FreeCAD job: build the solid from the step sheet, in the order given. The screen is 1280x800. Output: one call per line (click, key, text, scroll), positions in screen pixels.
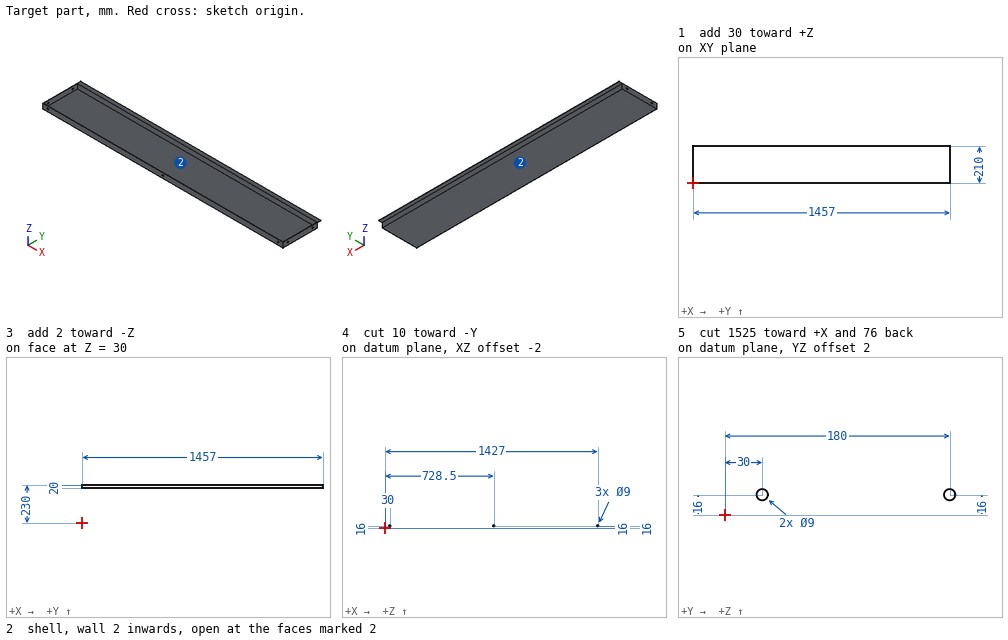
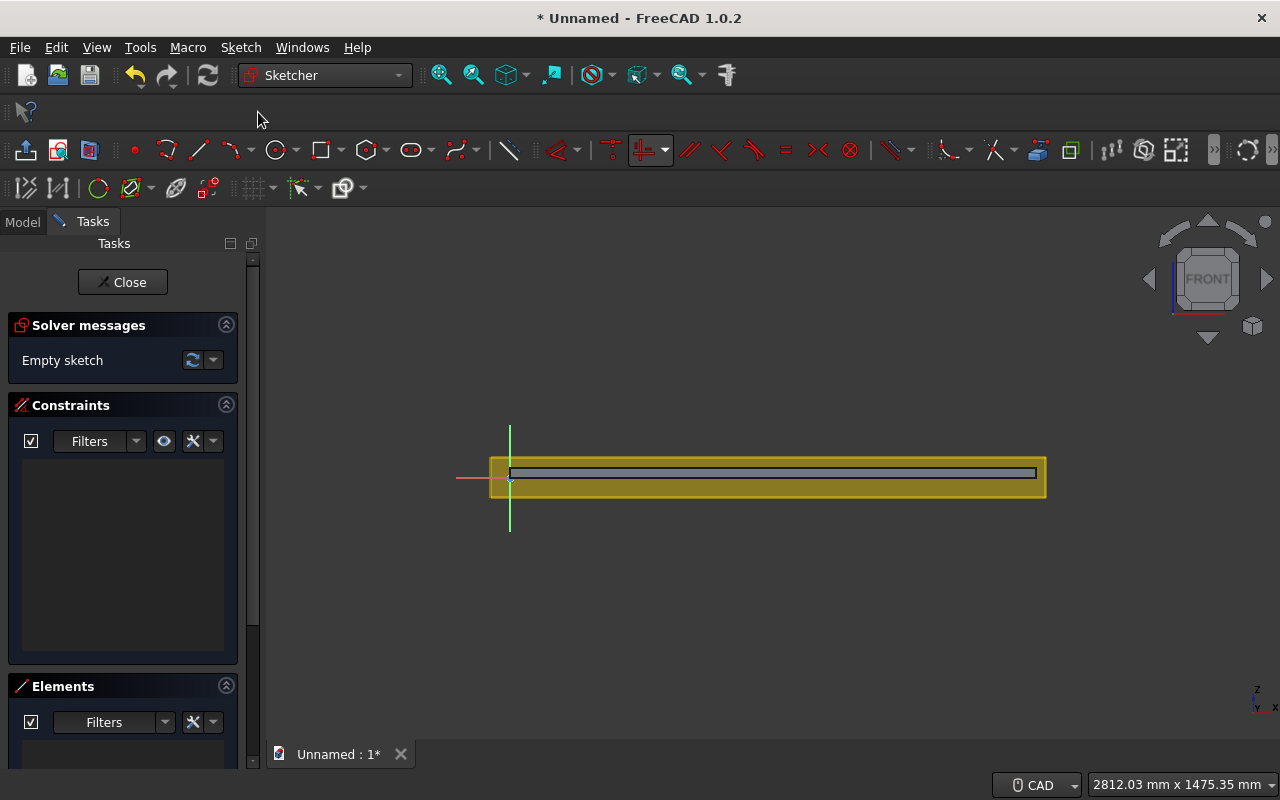
click(90, 150)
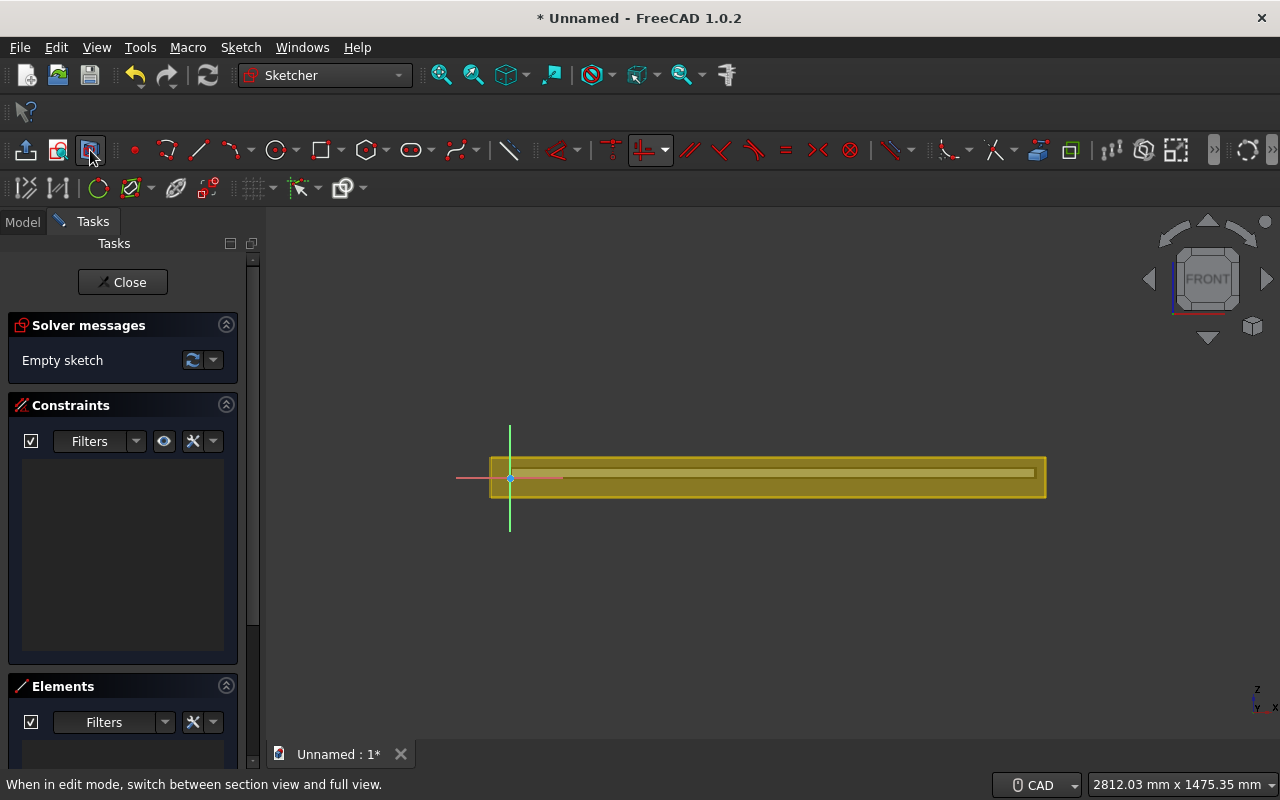
click(276, 150)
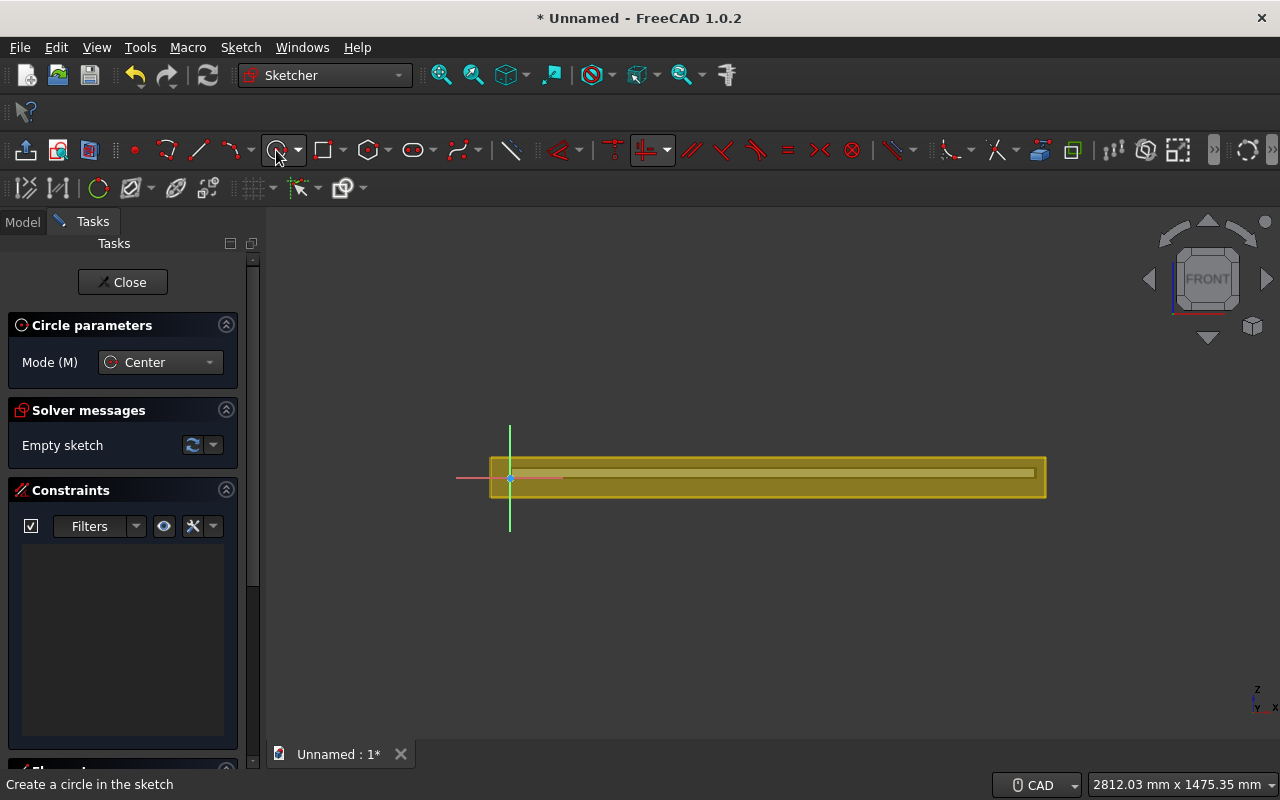
scroll(1025, 473, up, 14)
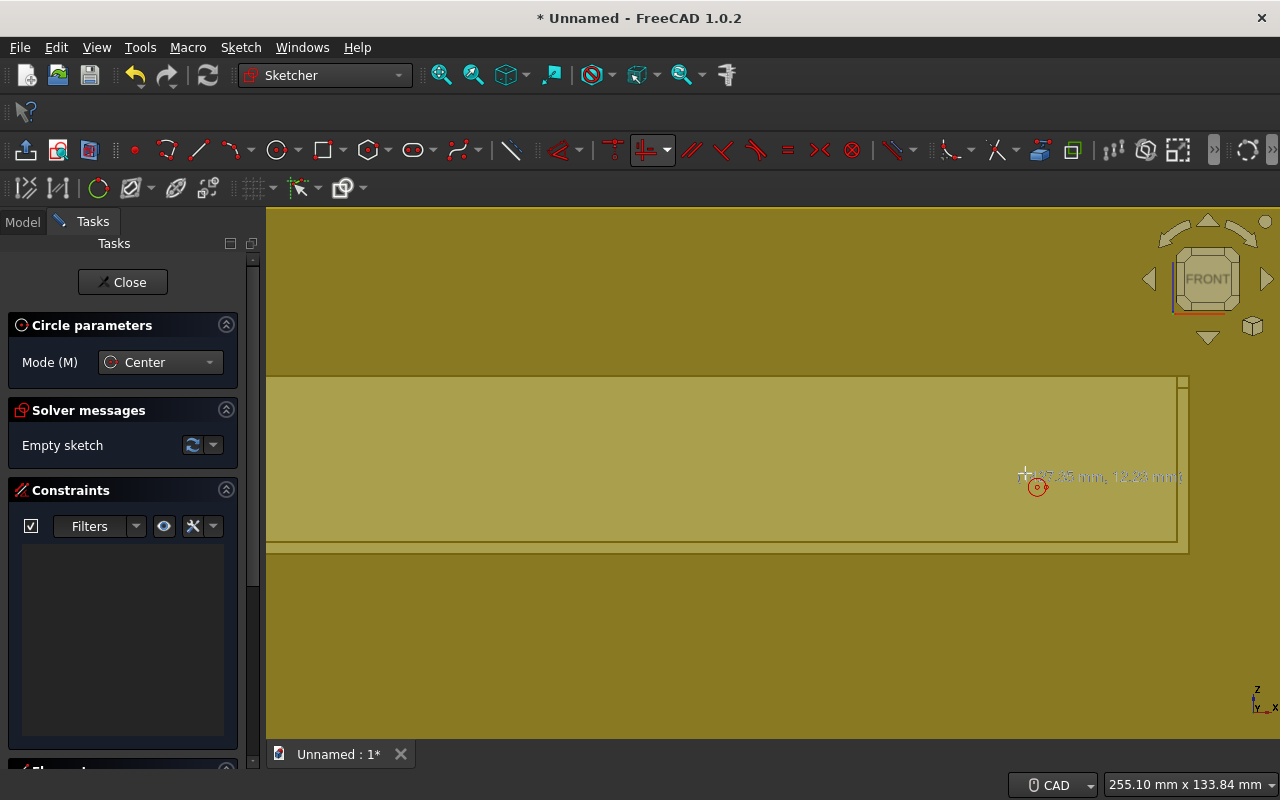
scroll(1018, 471, down, 13)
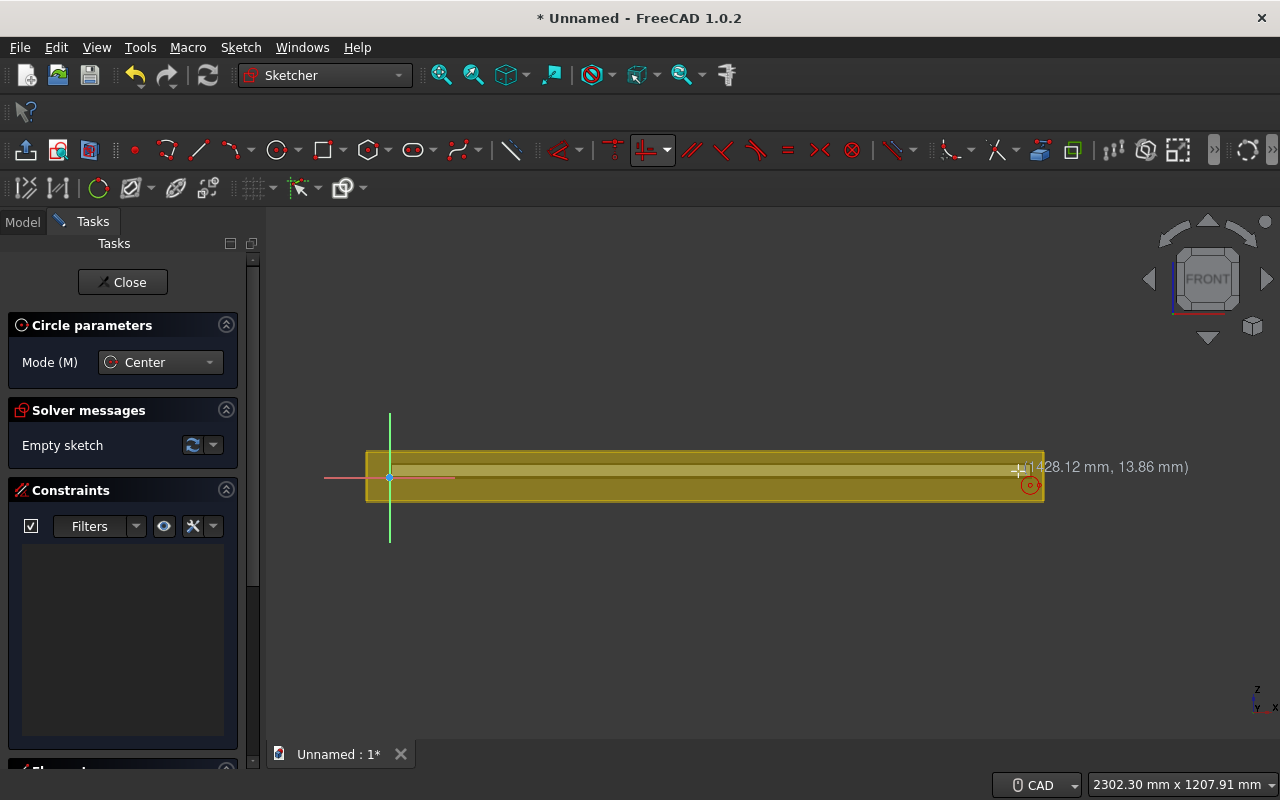
scroll(1018, 471, up, 5)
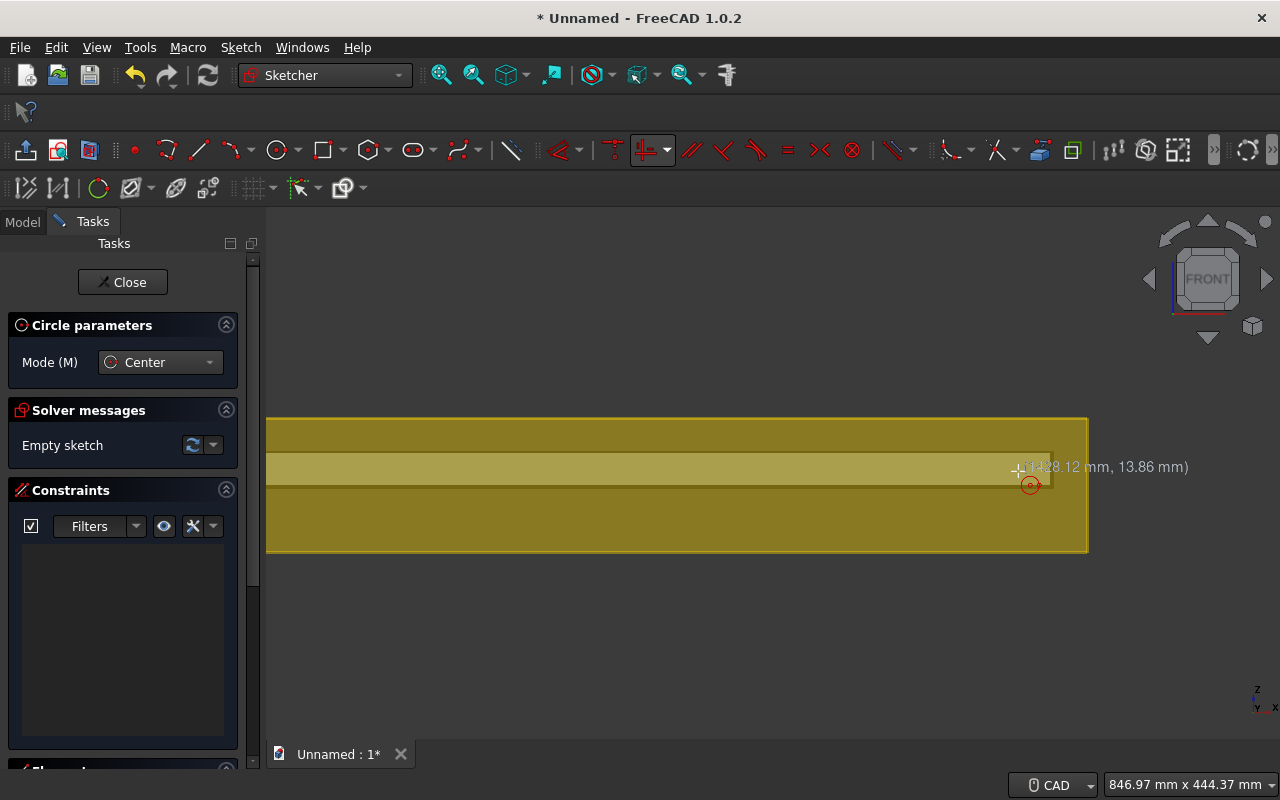
click(1017, 469)
move(1021, 465)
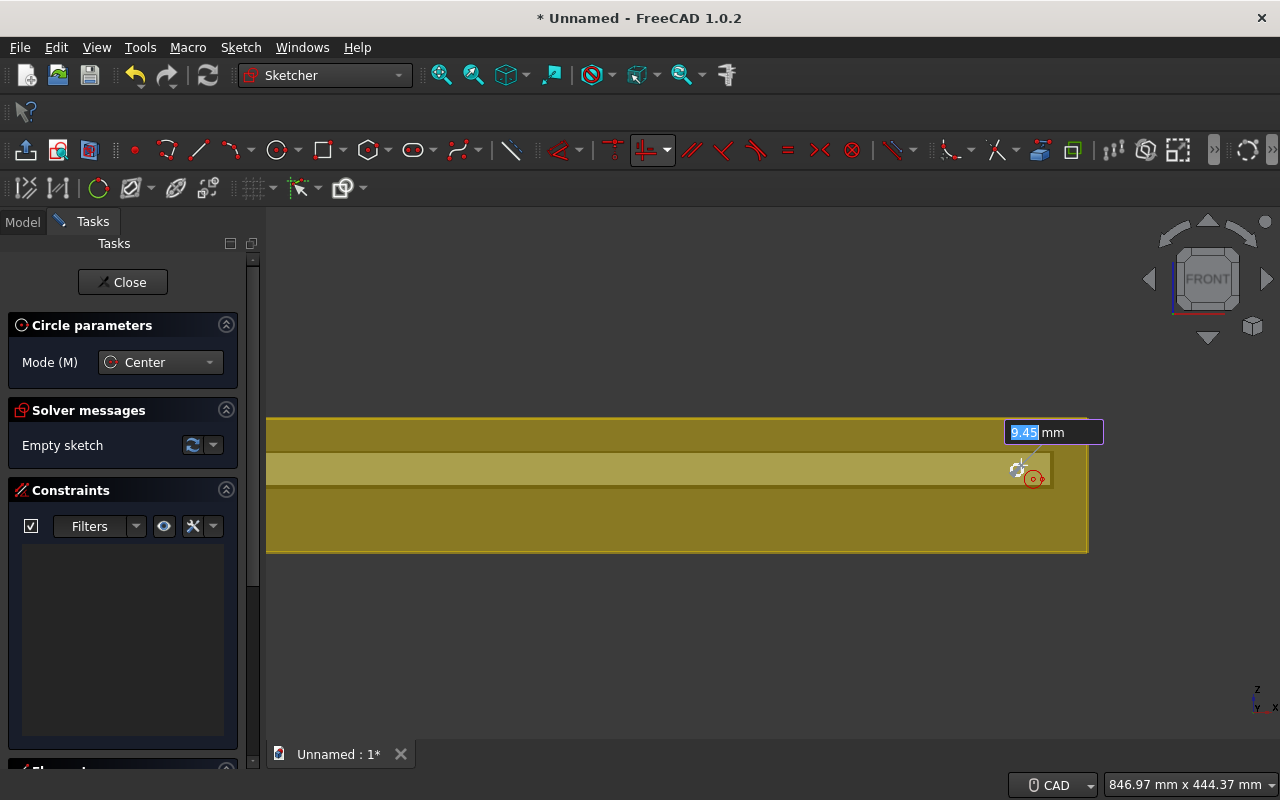
text(9)
key(Return)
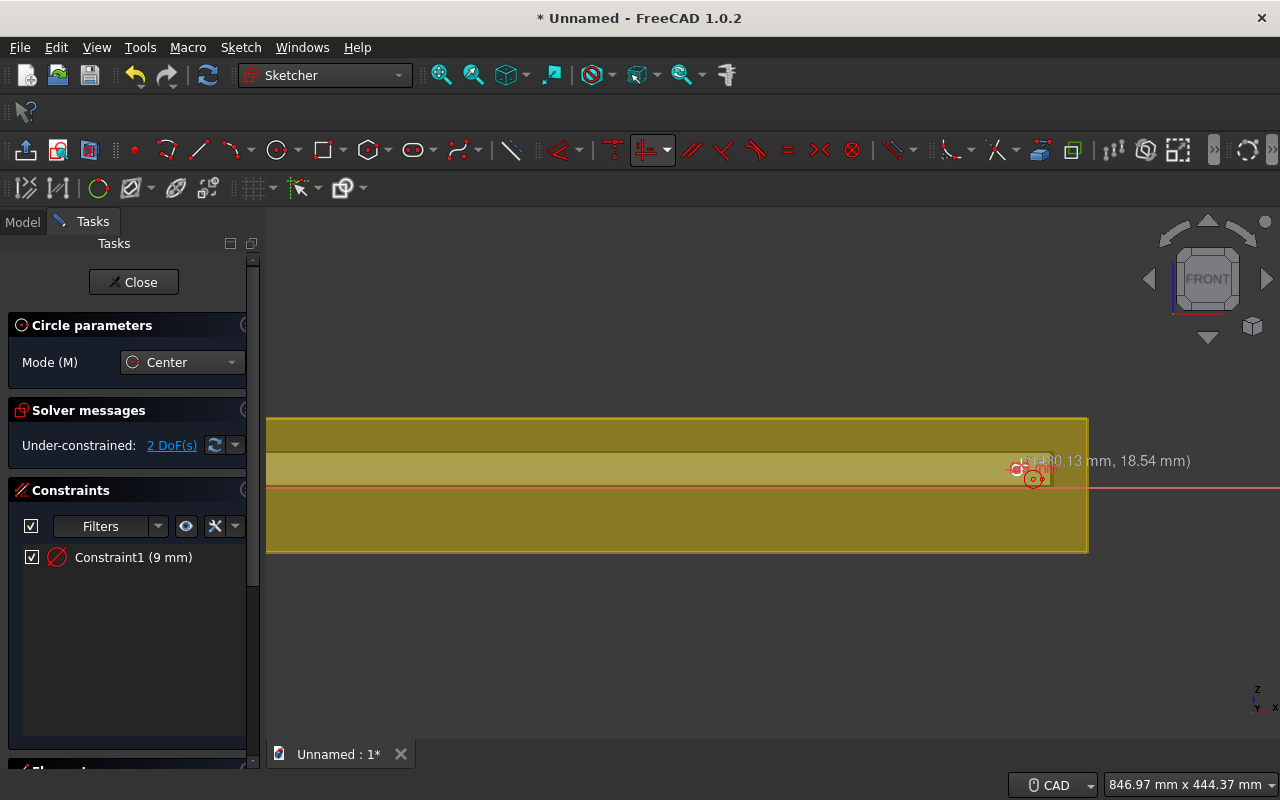
scroll(1018, 471, down, 5)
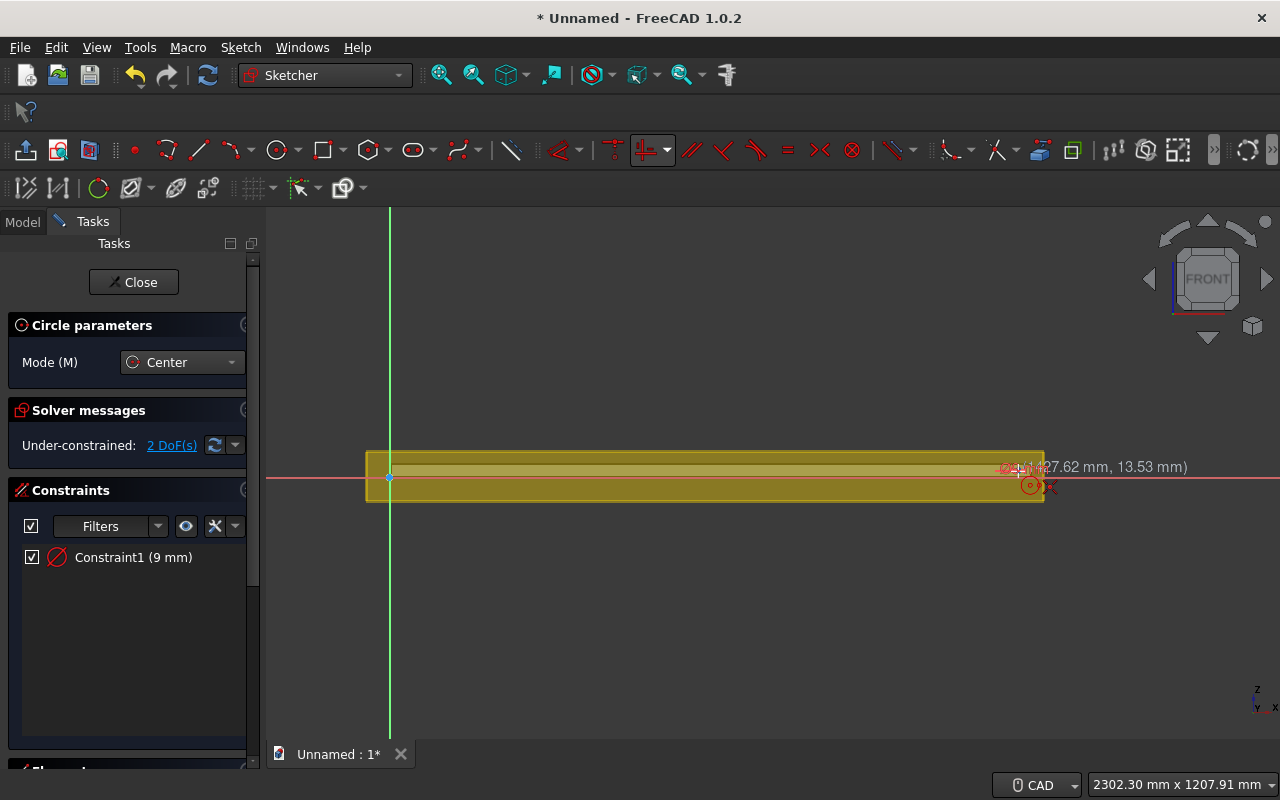
scroll(711, 471, up, 13)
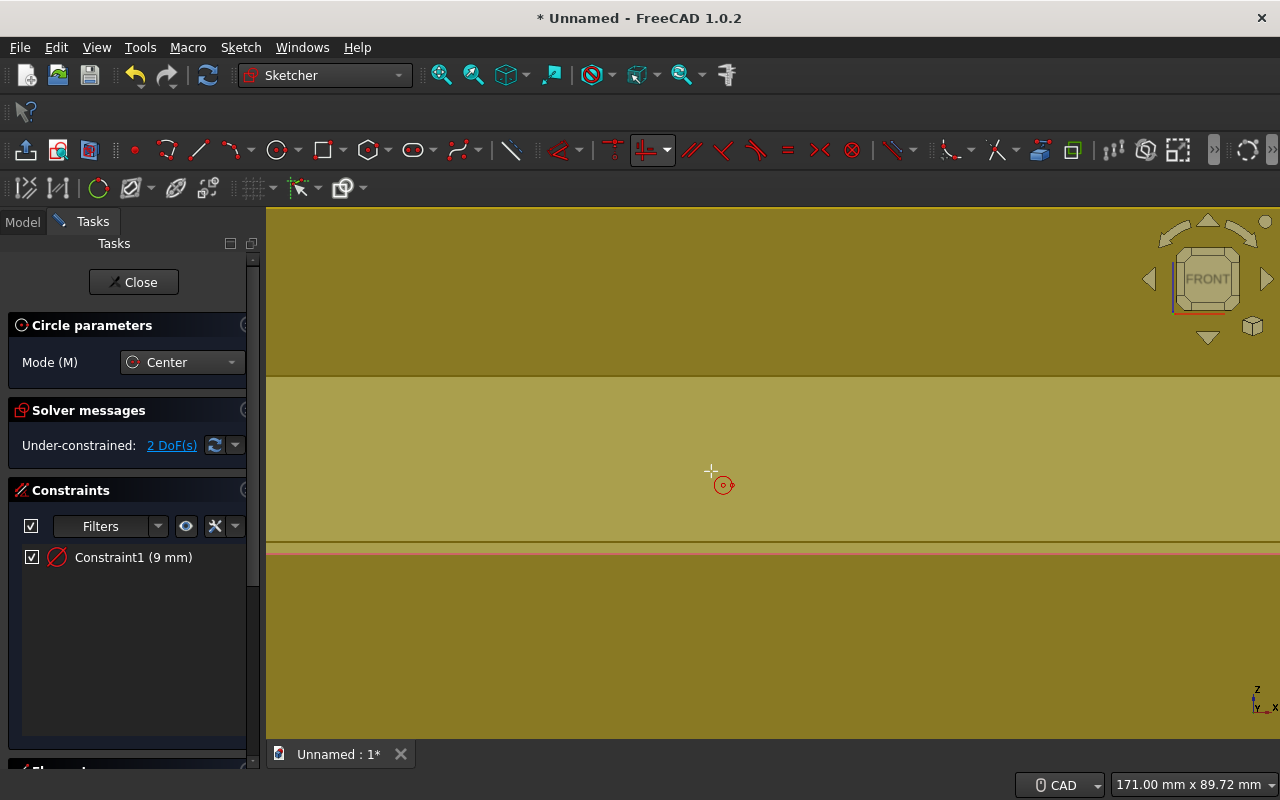
scroll(711, 471, down, 13)